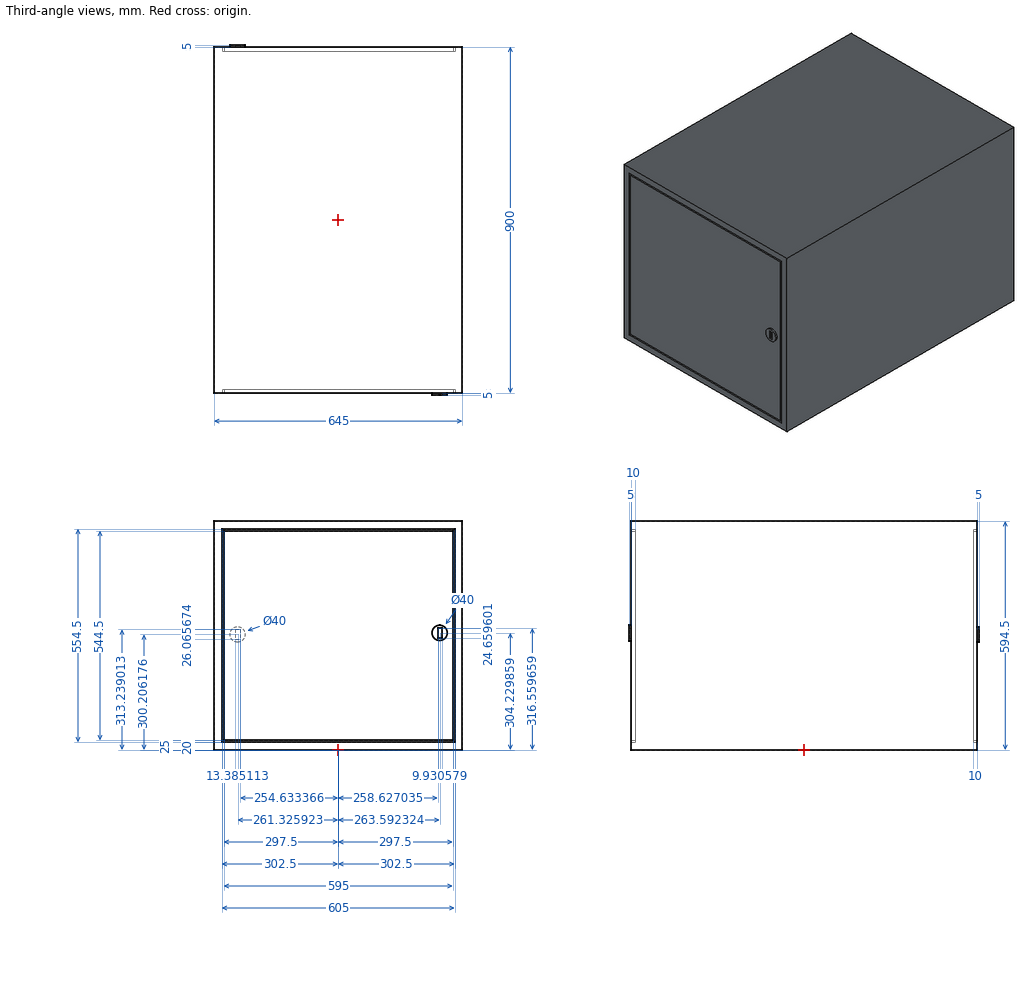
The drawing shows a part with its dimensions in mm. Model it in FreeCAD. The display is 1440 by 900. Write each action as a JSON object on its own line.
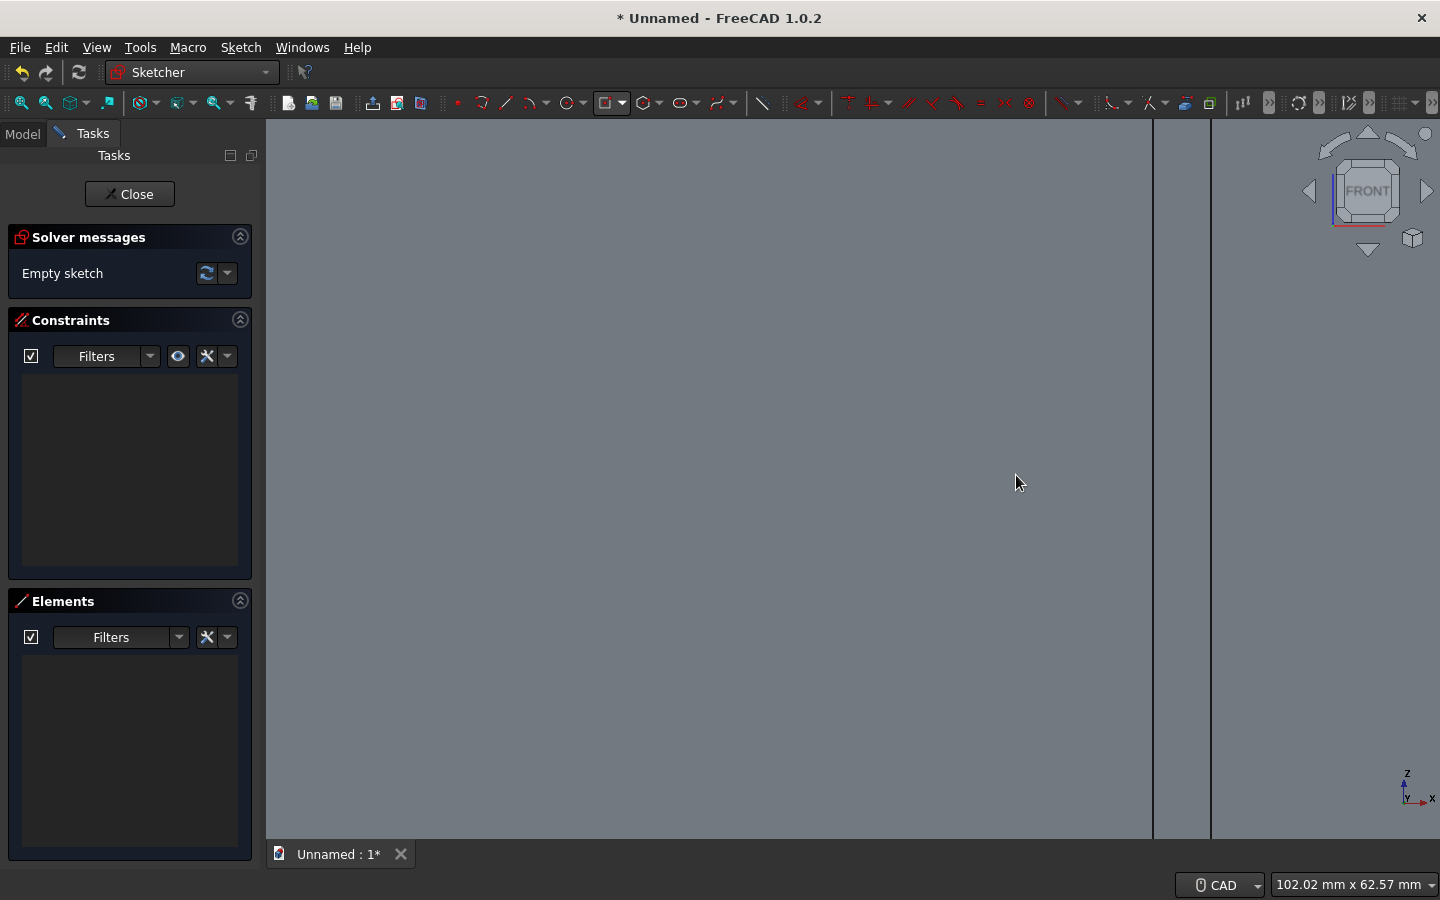
{"action": "key", "text": "g c"}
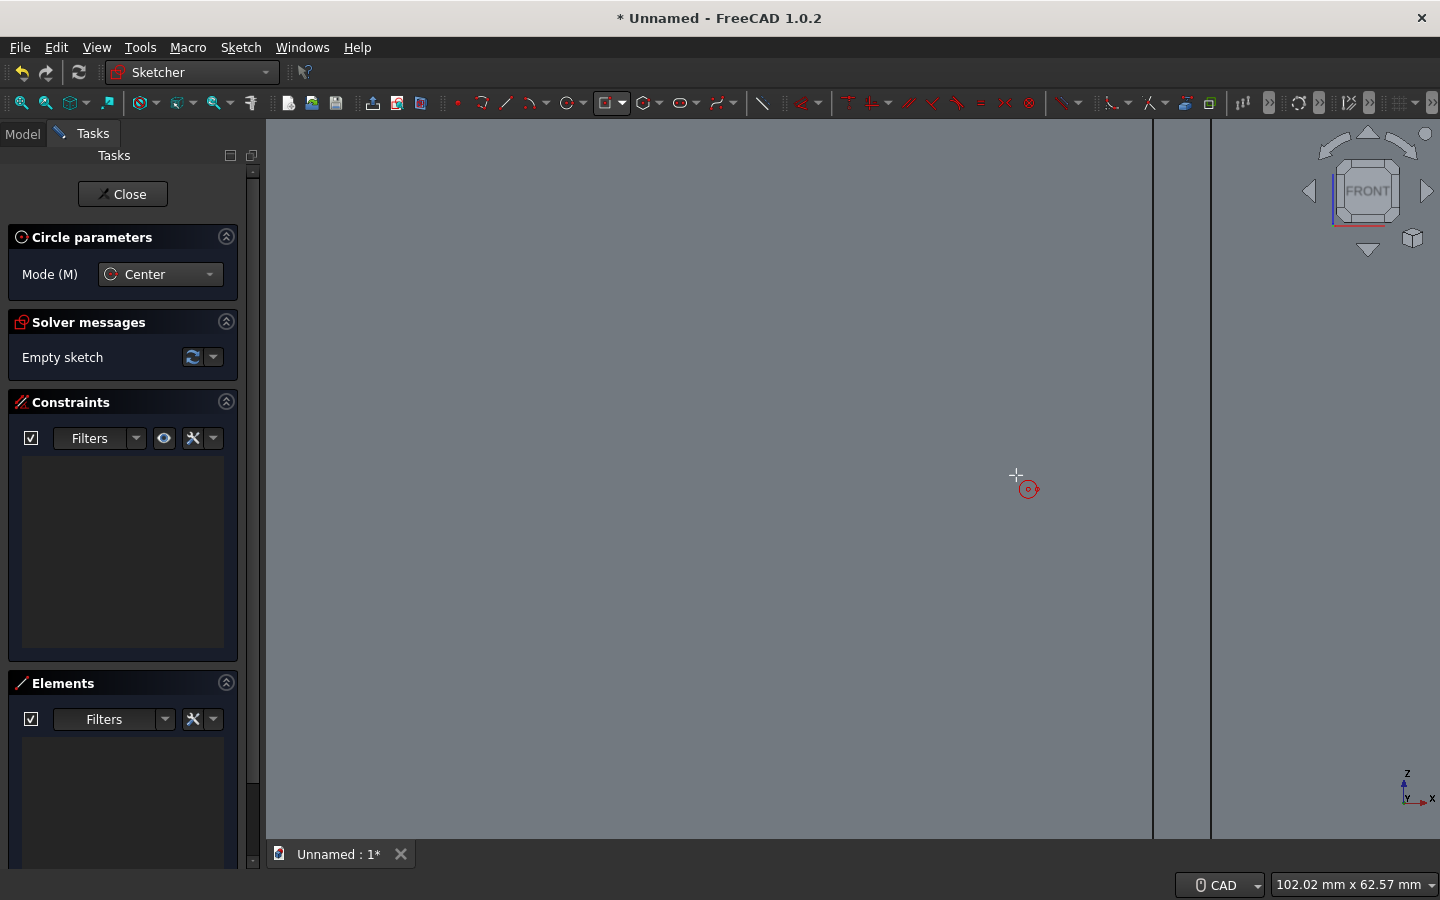
{"action": "left_click", "coordinate": [763, 466]}
{"action": "left_click", "coordinate": [926, 303]}
{"action": "key", "text": "Escape"}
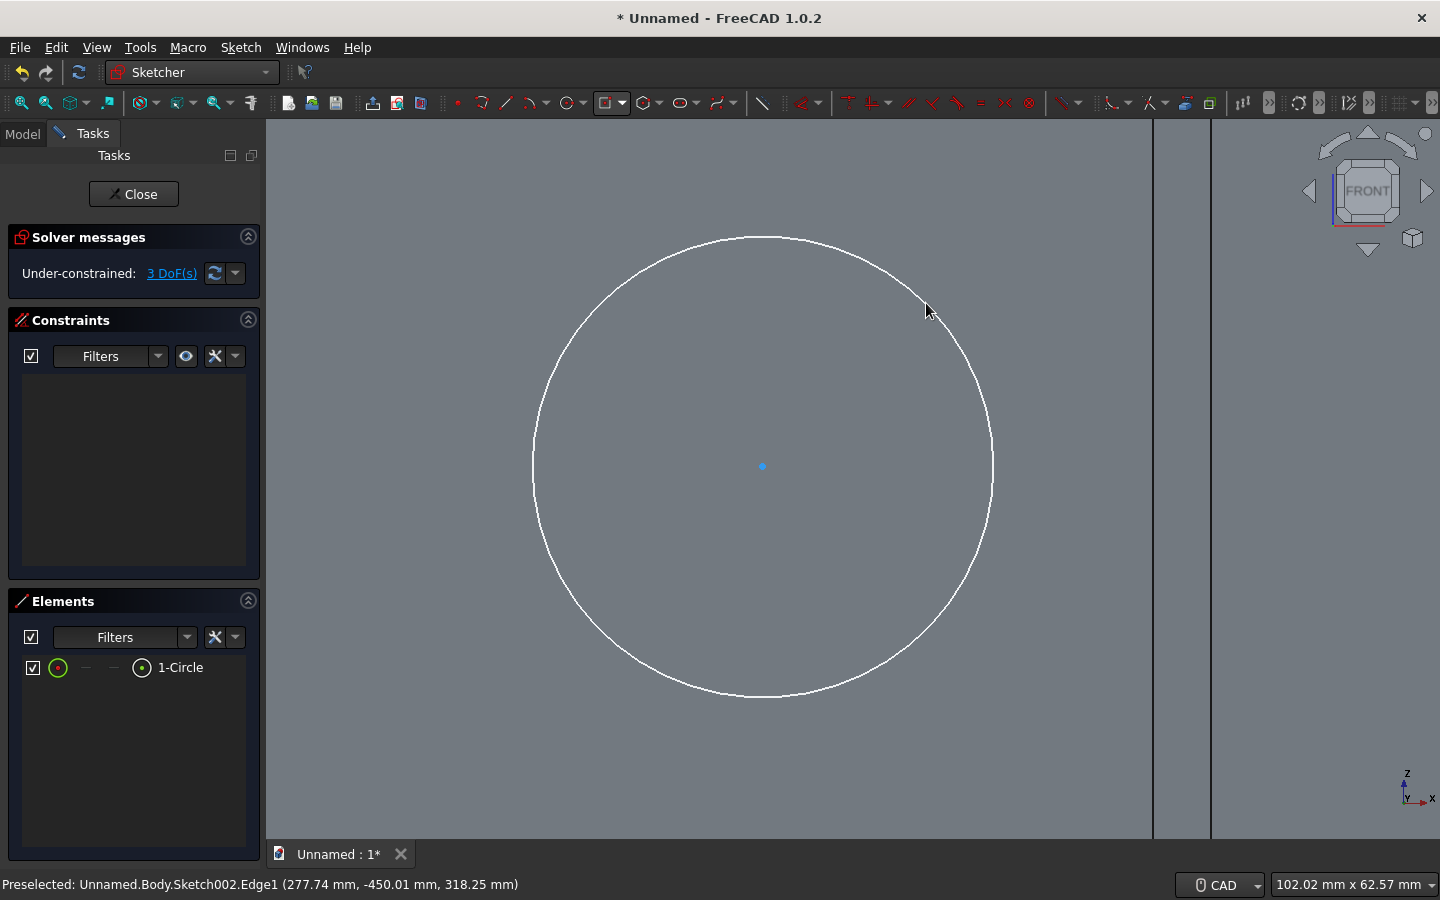
{"action": "key", "text": "d"}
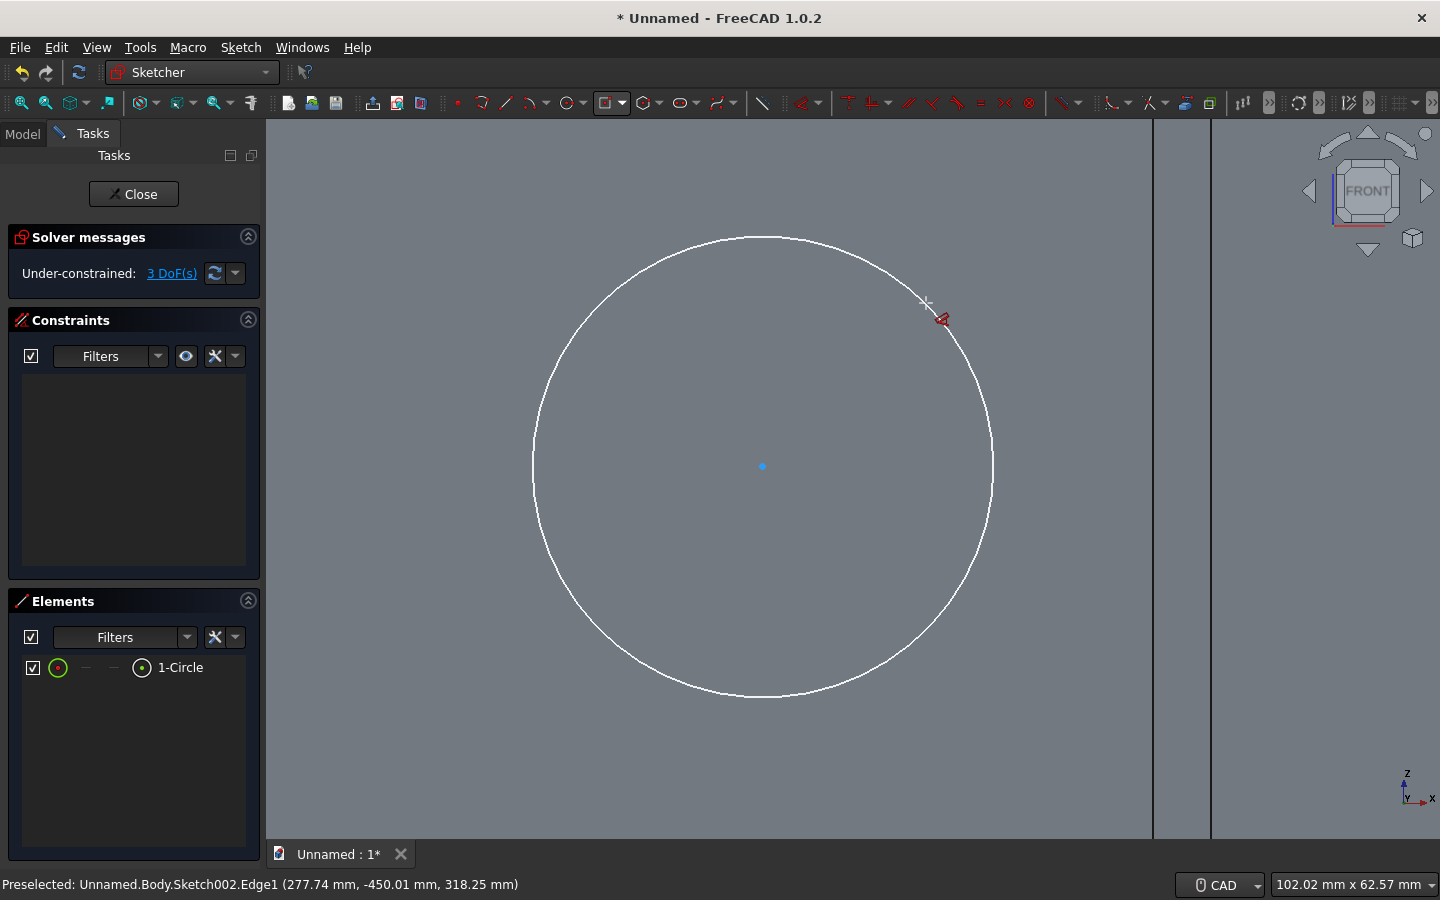
{"action": "left_click", "coordinate": [925, 303]}
{"action": "left_click", "coordinate": [947, 280]}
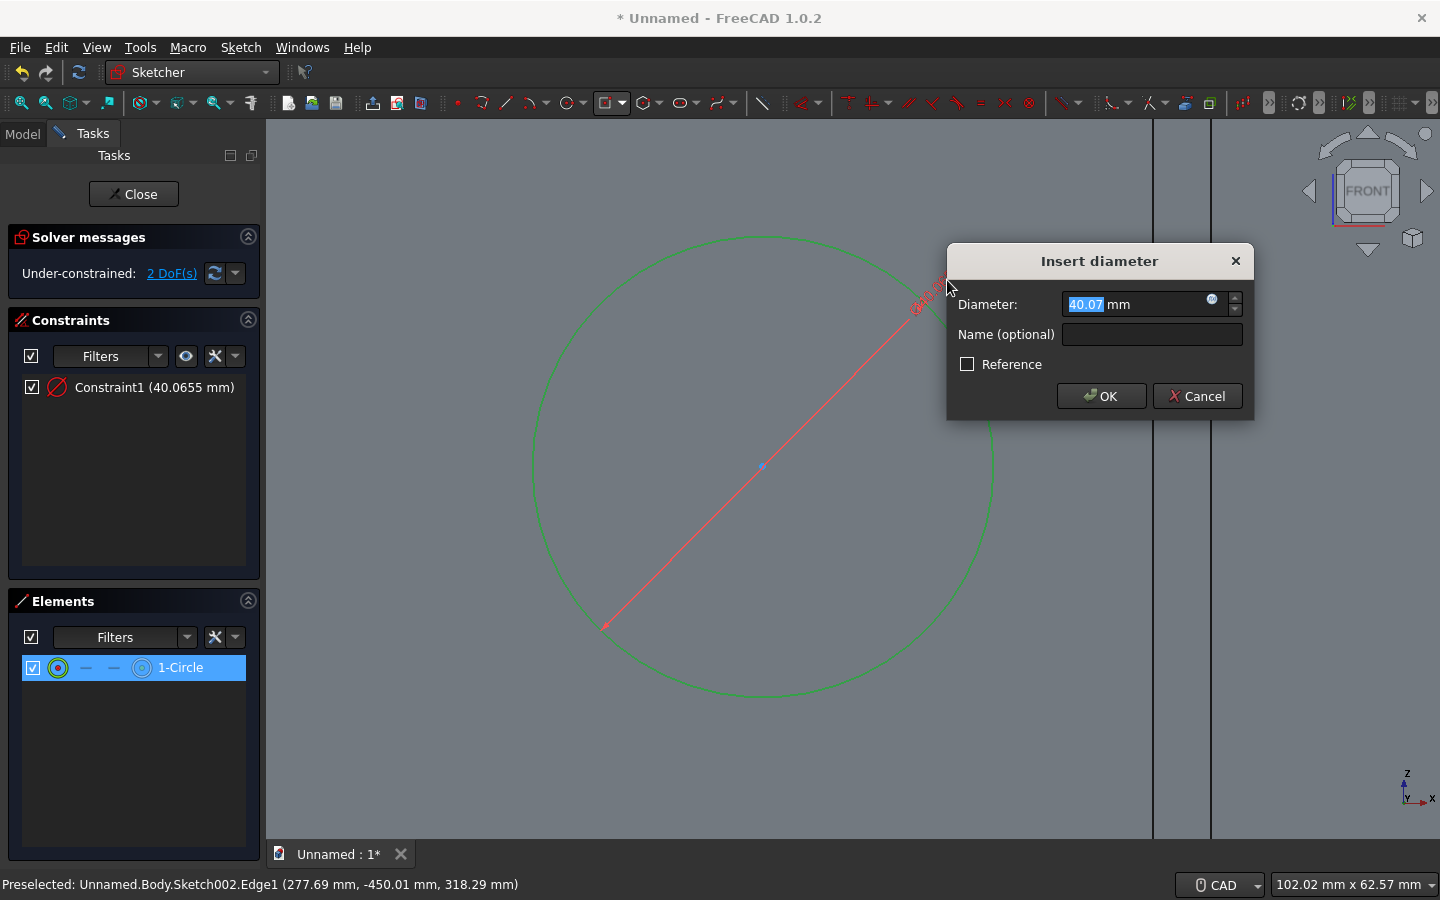
{"action": "type", "text": "40"}
{"action": "key", "text": "Return"}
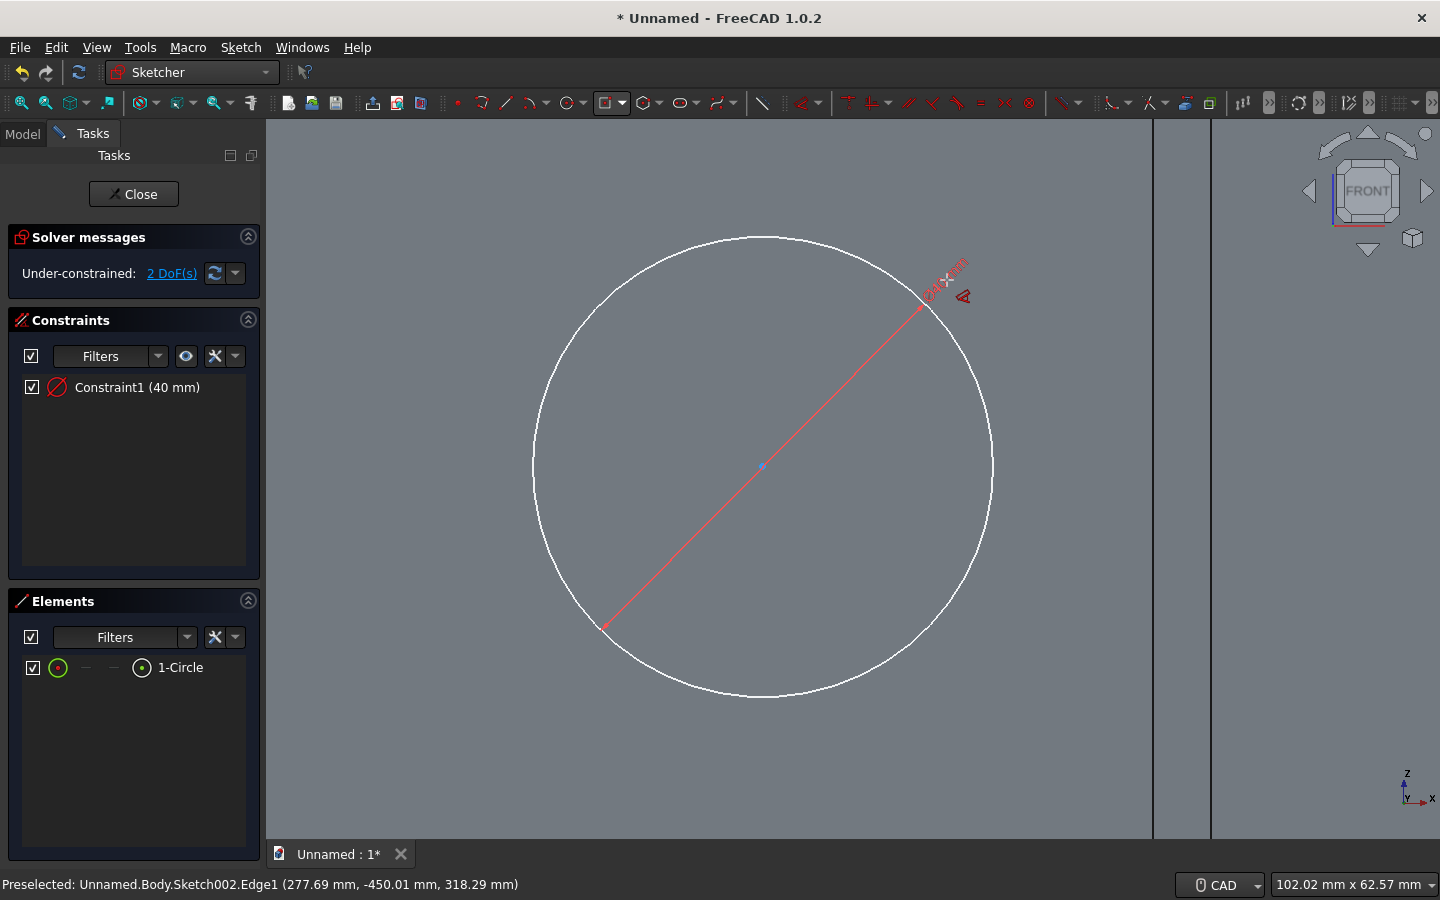
{"action": "left_click", "coordinate": [763, 467]}
{"action": "left_click", "coordinate": [421, 433]}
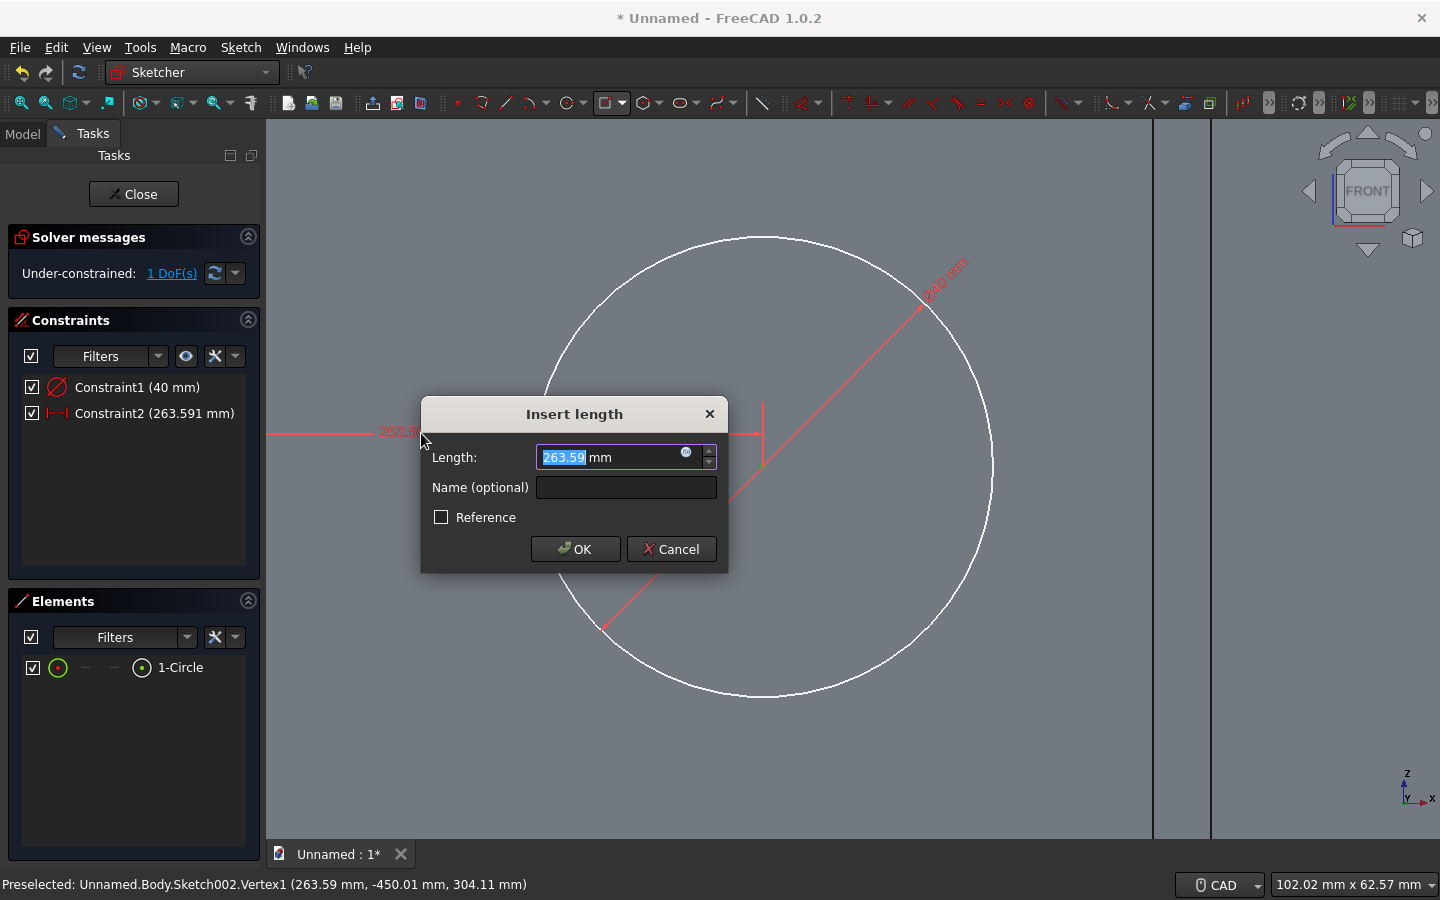
{"action": "type", "text": "263.592324"}
{"action": "key", "text": "Return"}